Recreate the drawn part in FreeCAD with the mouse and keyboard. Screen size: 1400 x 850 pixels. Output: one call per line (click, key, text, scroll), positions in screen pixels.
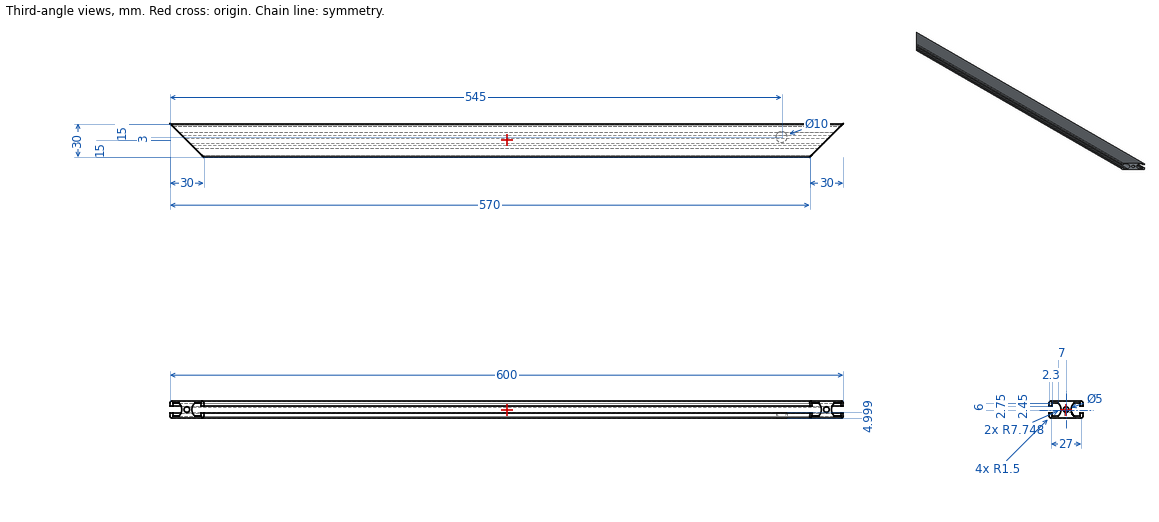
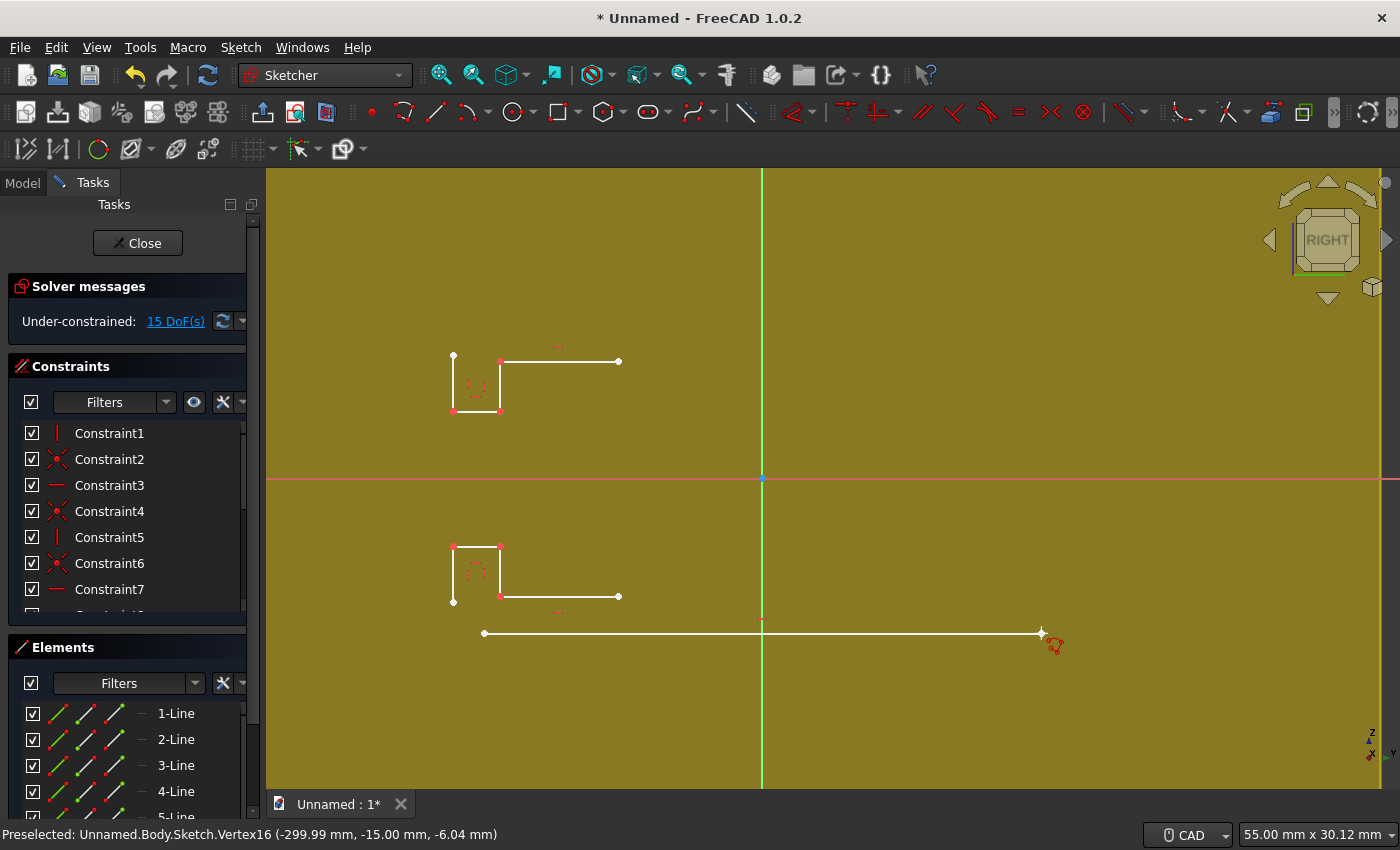
click(1071, 602)
click(1071, 546)
click(1024, 546)
click(1024, 596)
click(906, 596)
right_click(906, 596)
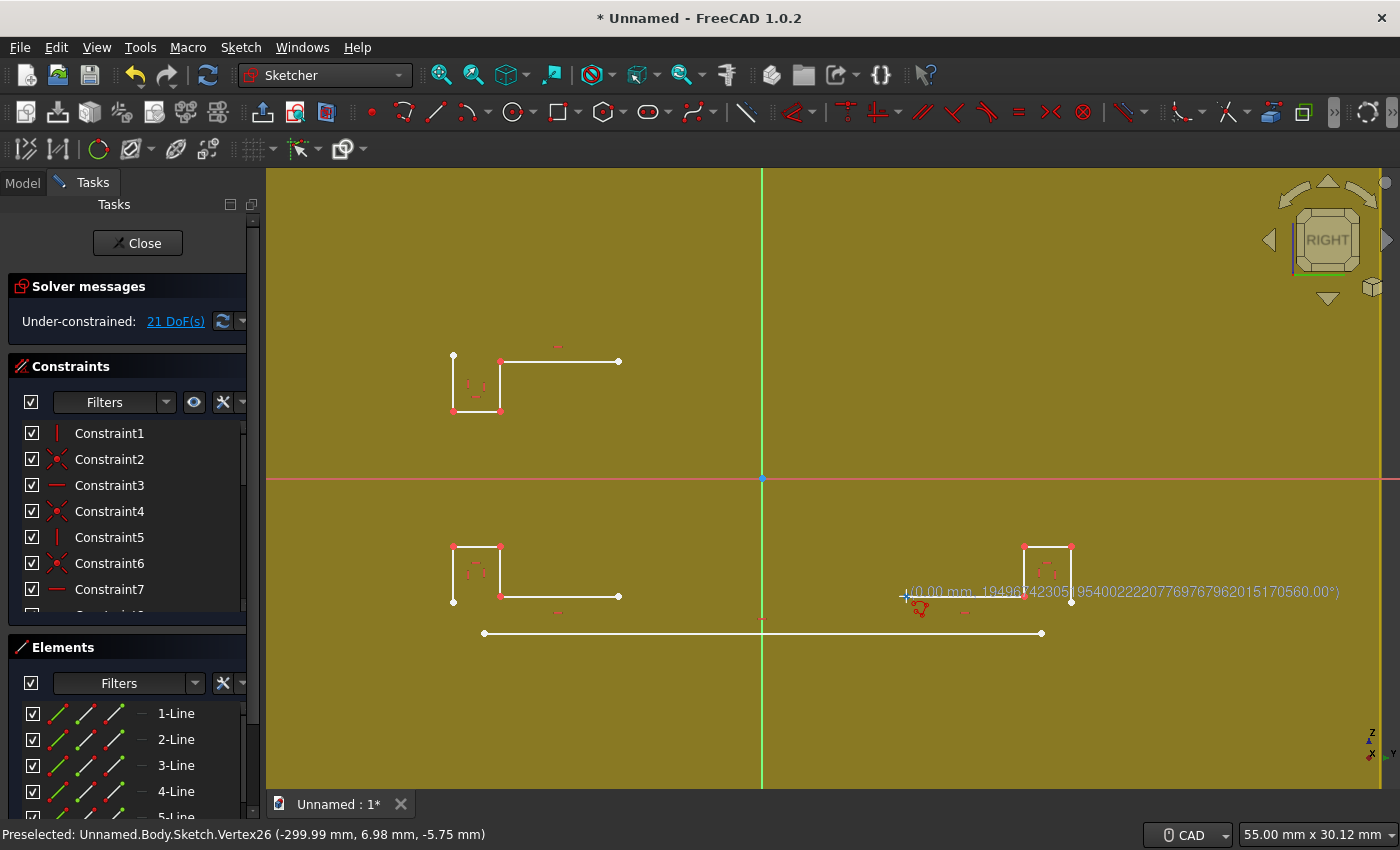
click(906, 361)
click(1024, 361)
click(1024, 411)
click(1071, 411)
click(1071, 355)
right_click(1071, 355)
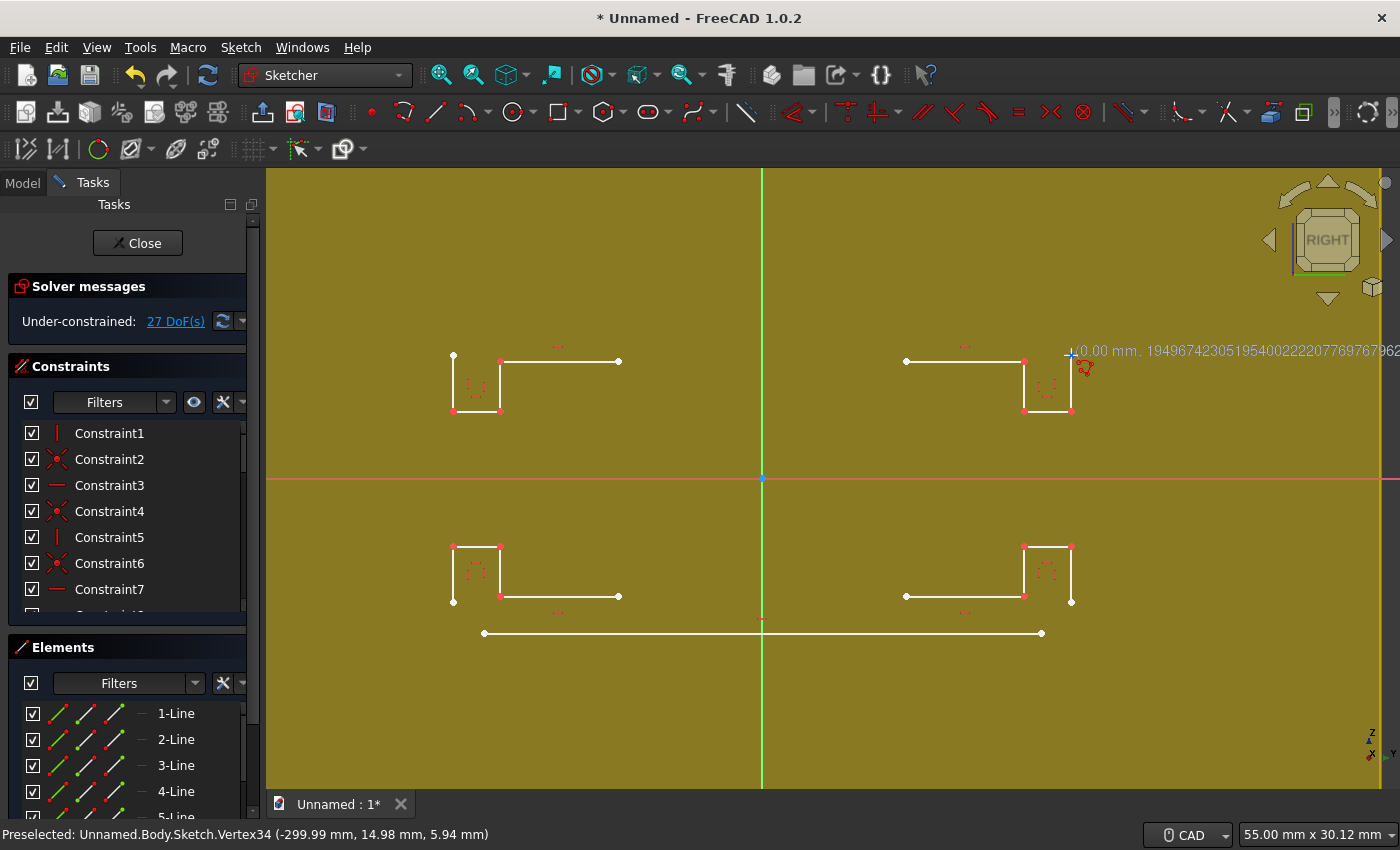
key(g)
key(l)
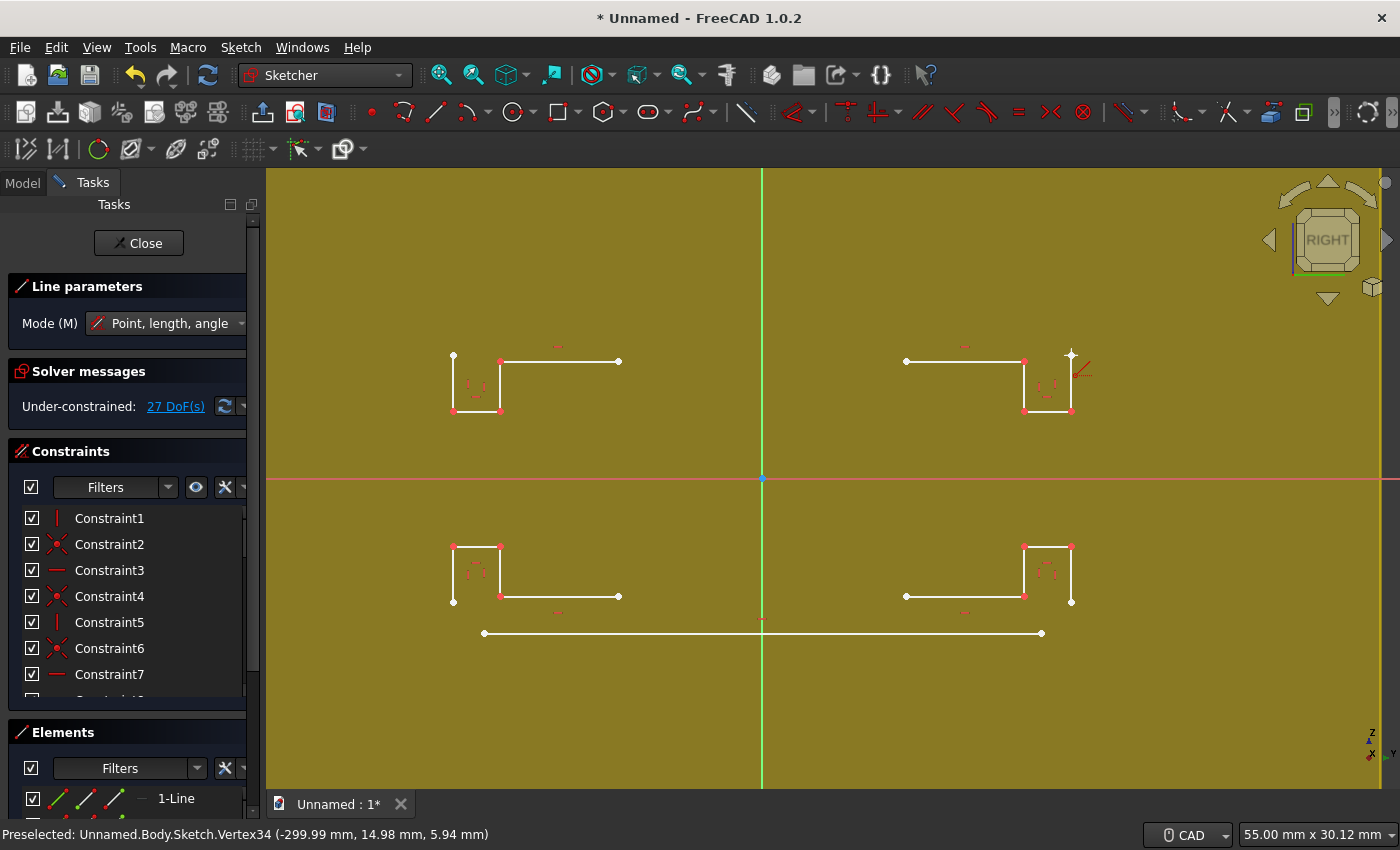
click(1041, 324)
click(484, 324)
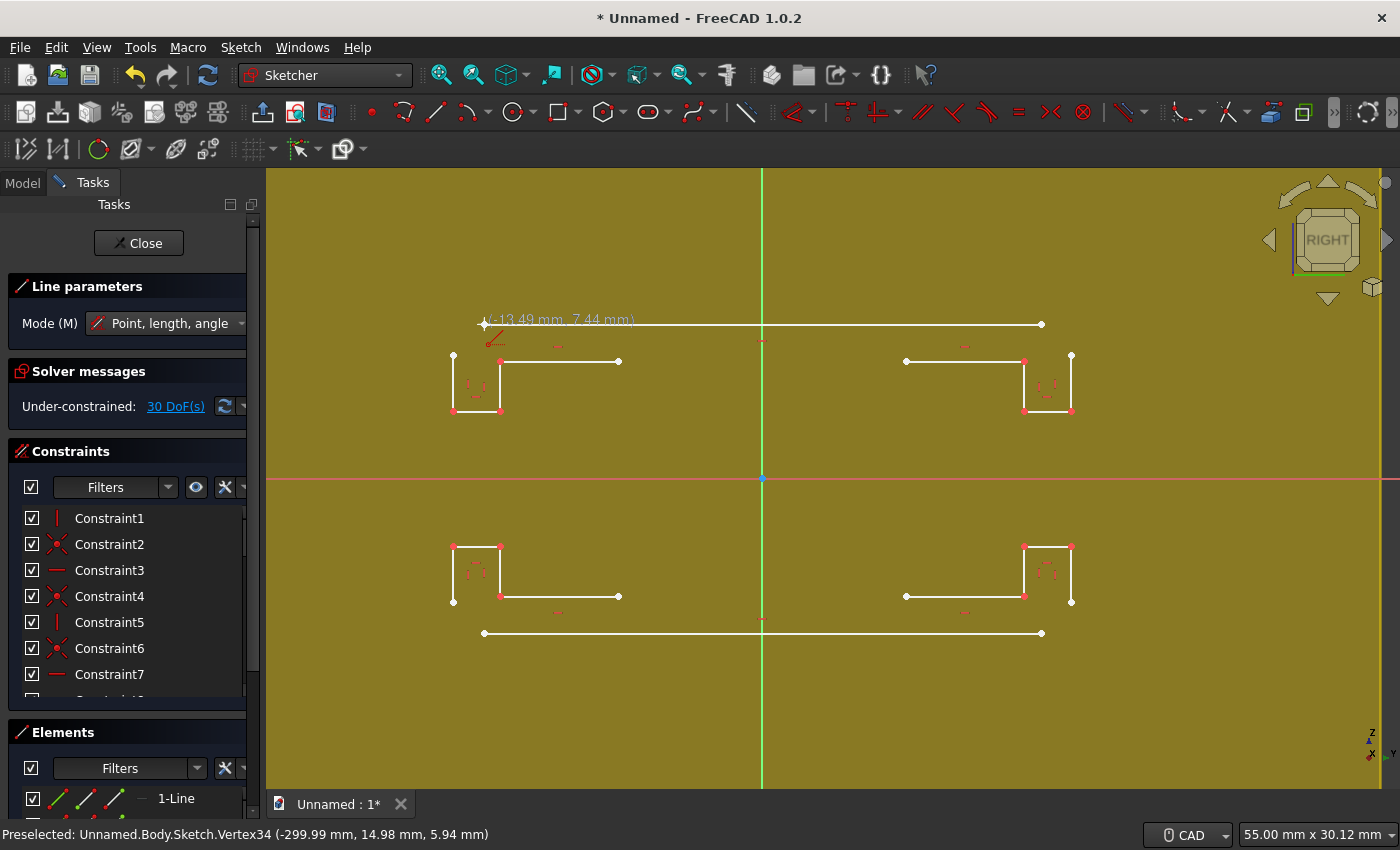
key(g)
key(3)
key(a)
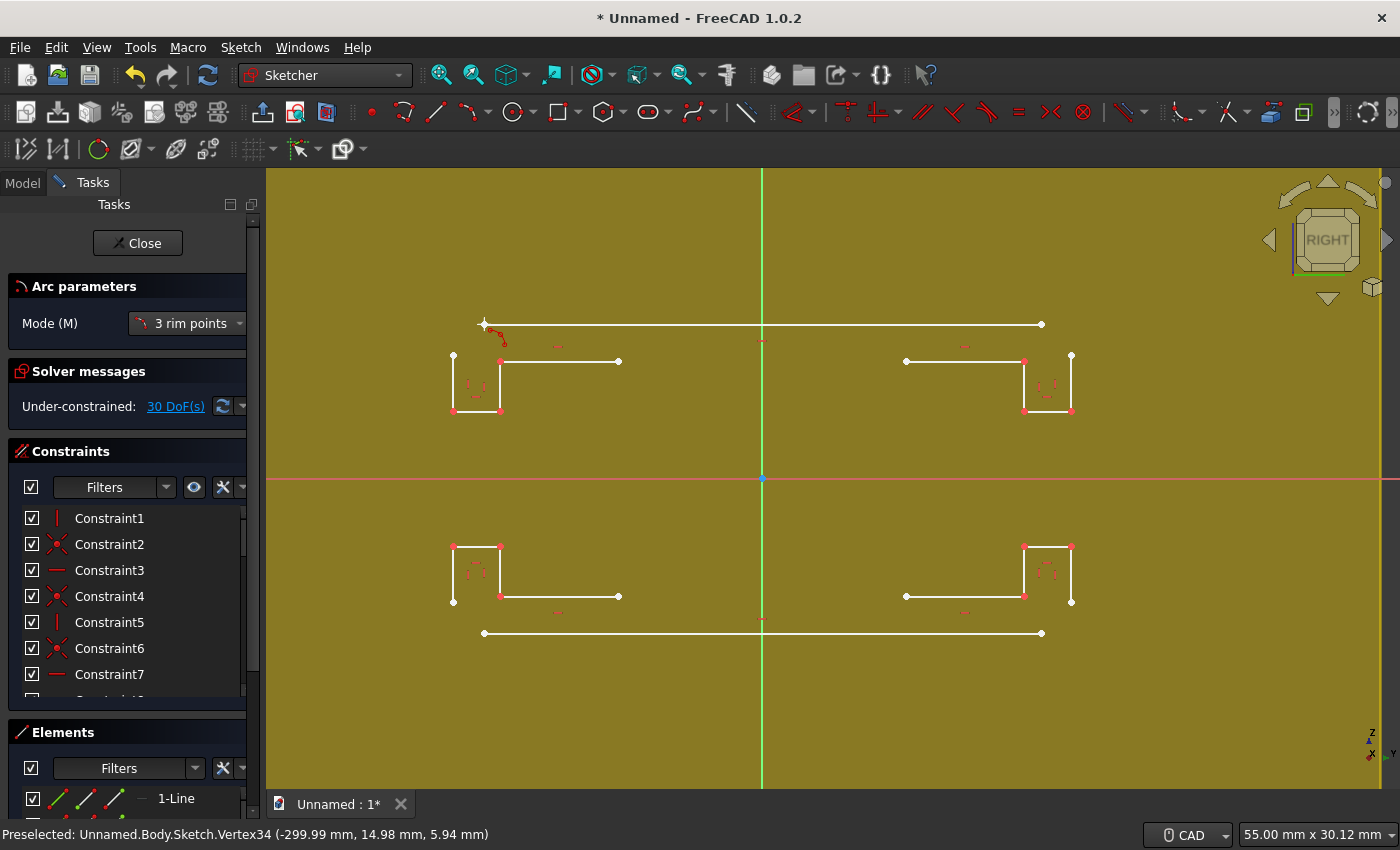
click(618, 362)
click(618, 597)
click(667, 505)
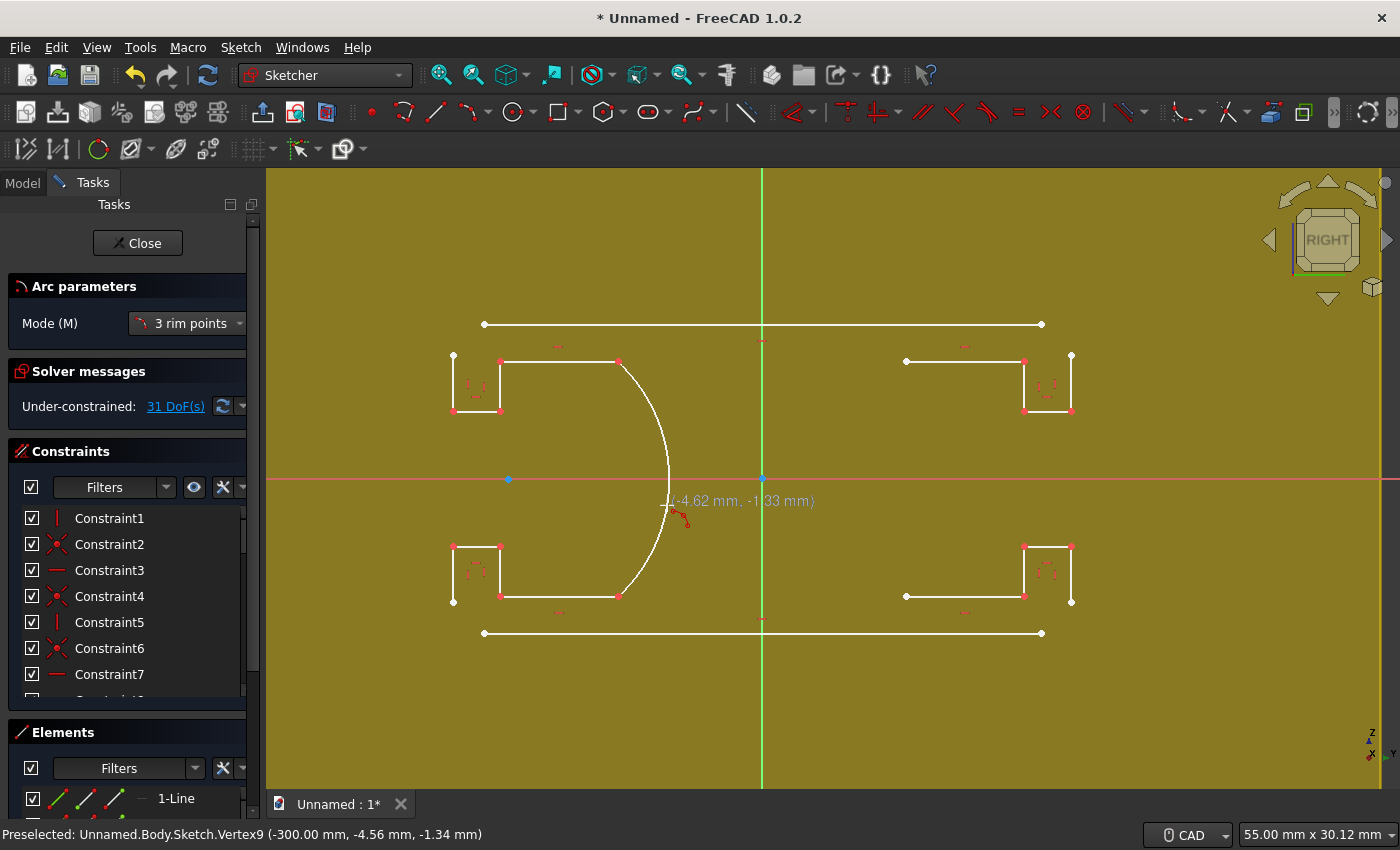
click(453, 603)
click(484, 634)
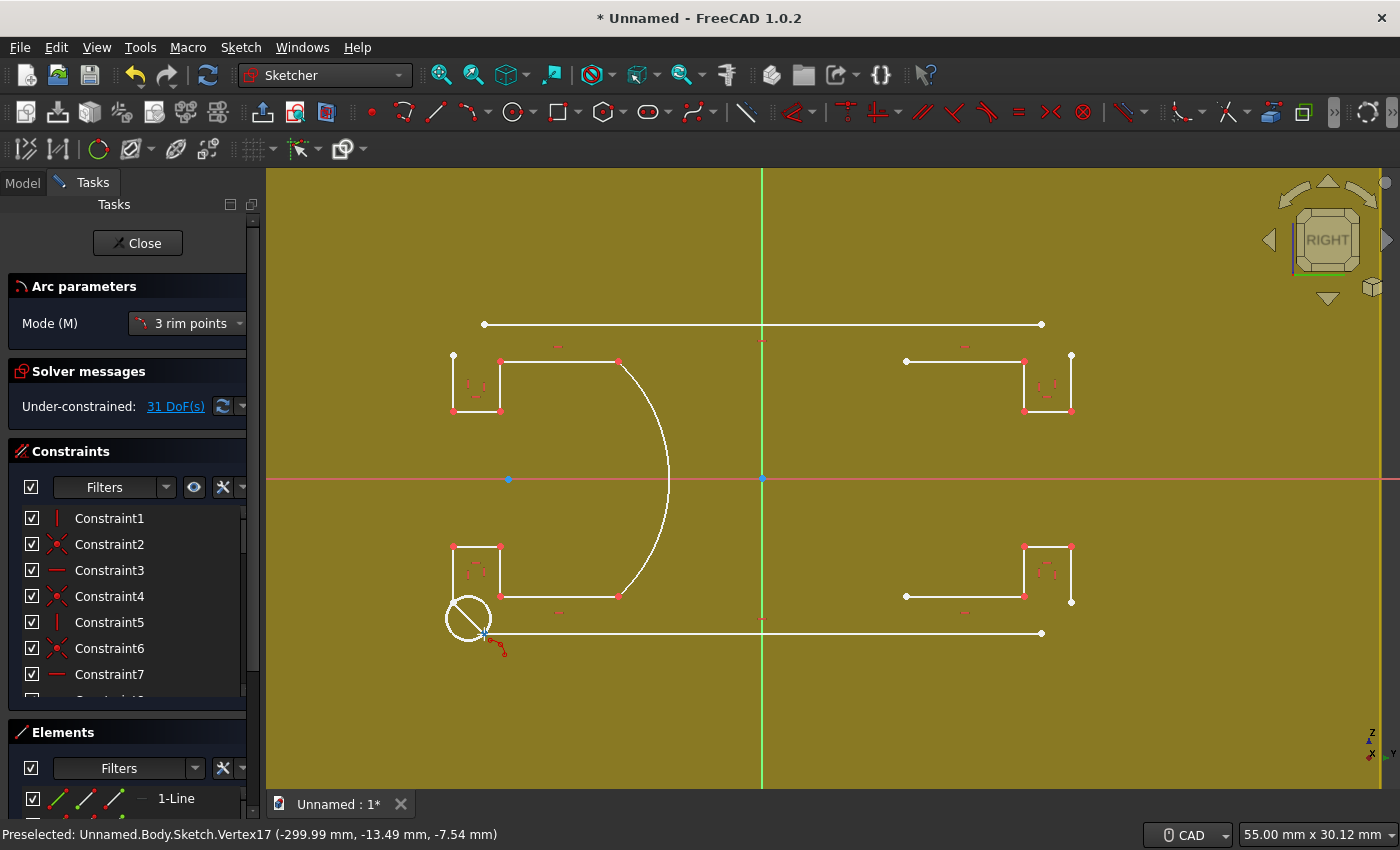
scroll(462, 624, up, 3)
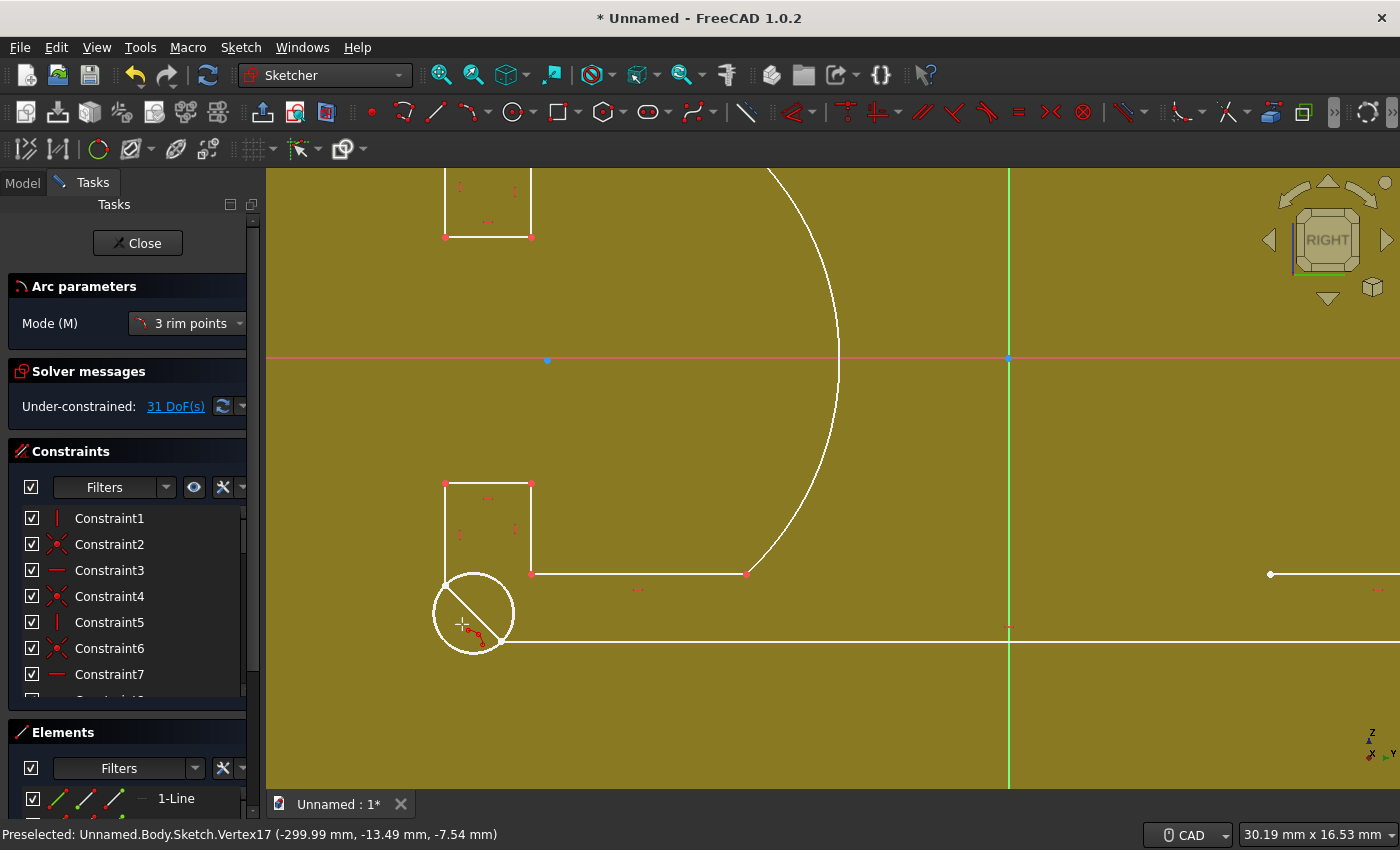
click(462, 624)